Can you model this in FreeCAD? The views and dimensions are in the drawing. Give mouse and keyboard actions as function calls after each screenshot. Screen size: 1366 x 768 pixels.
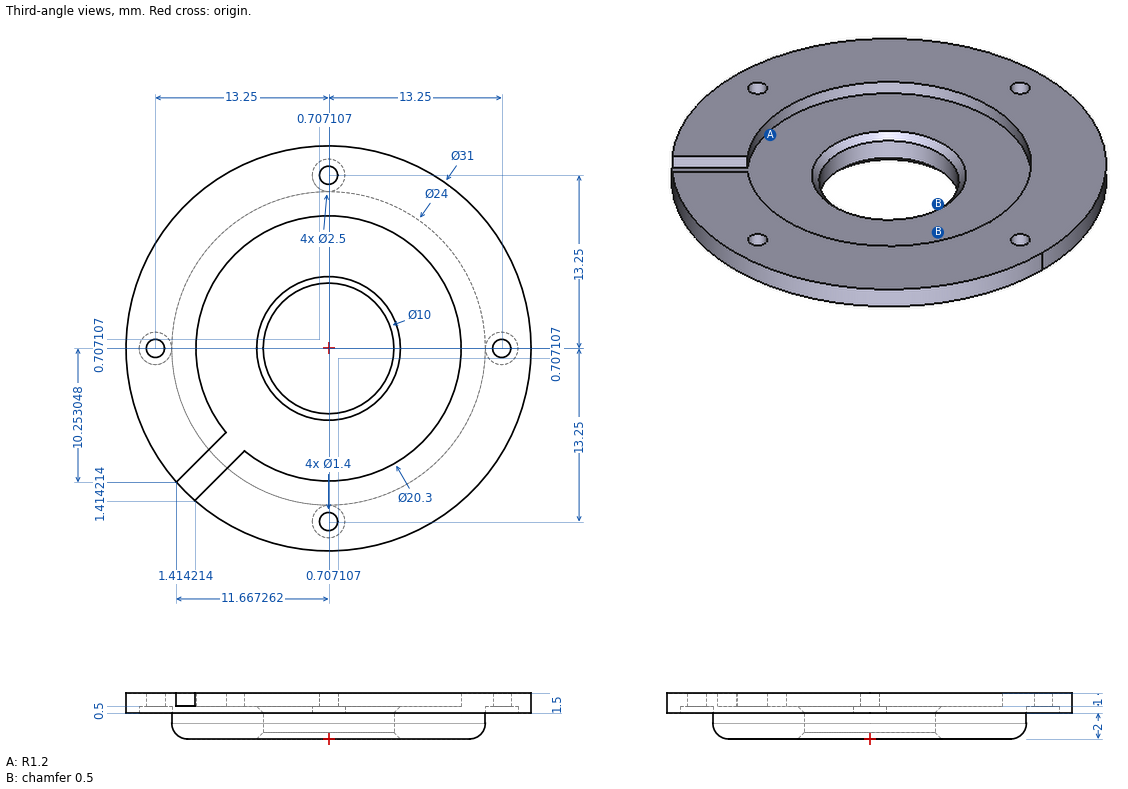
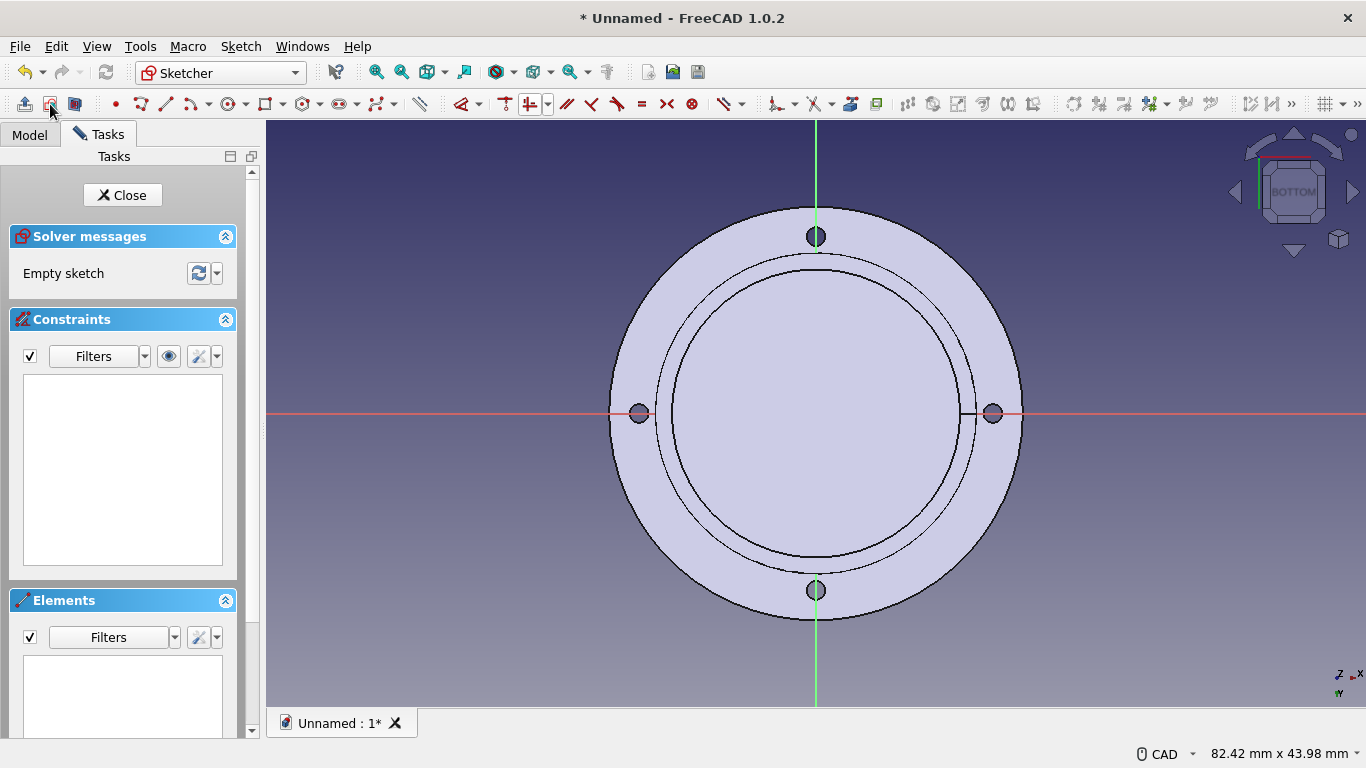
click(228, 104)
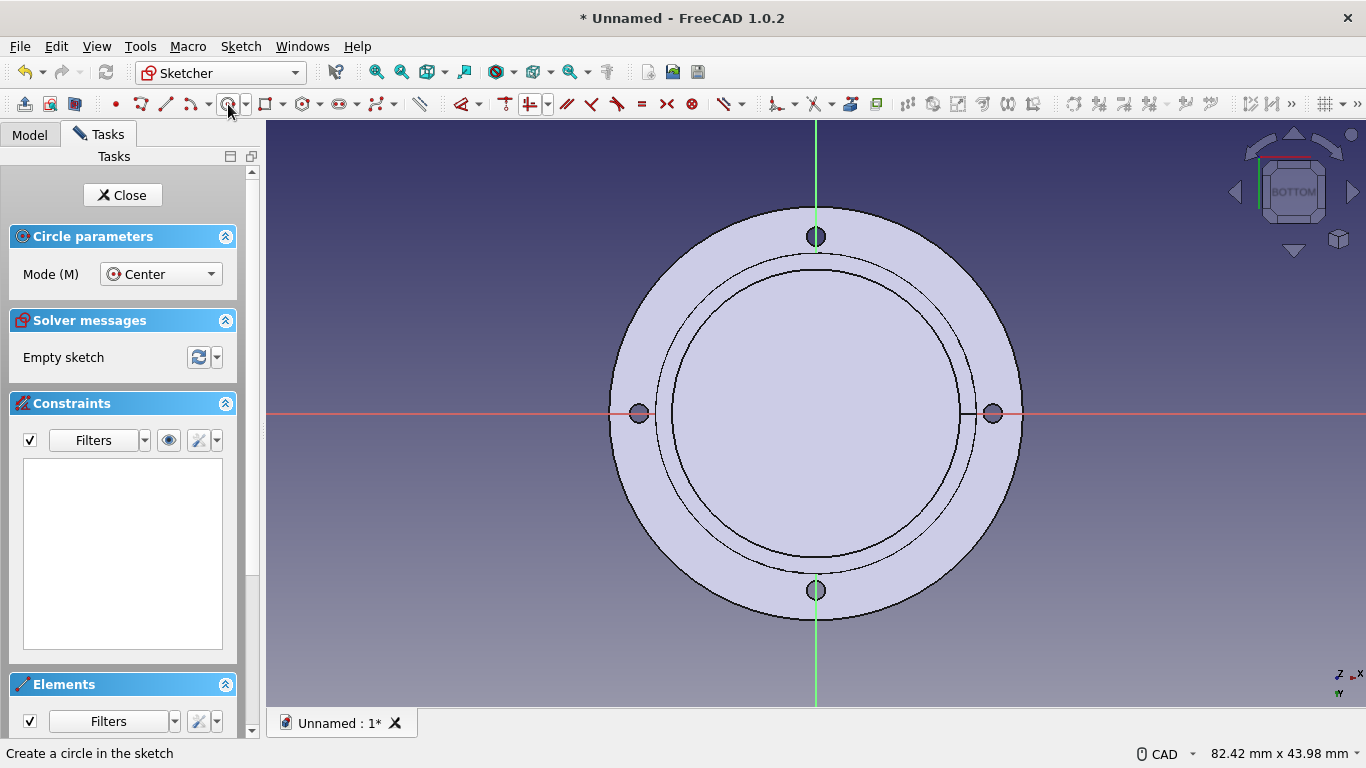
scroll(816, 590, up, 2)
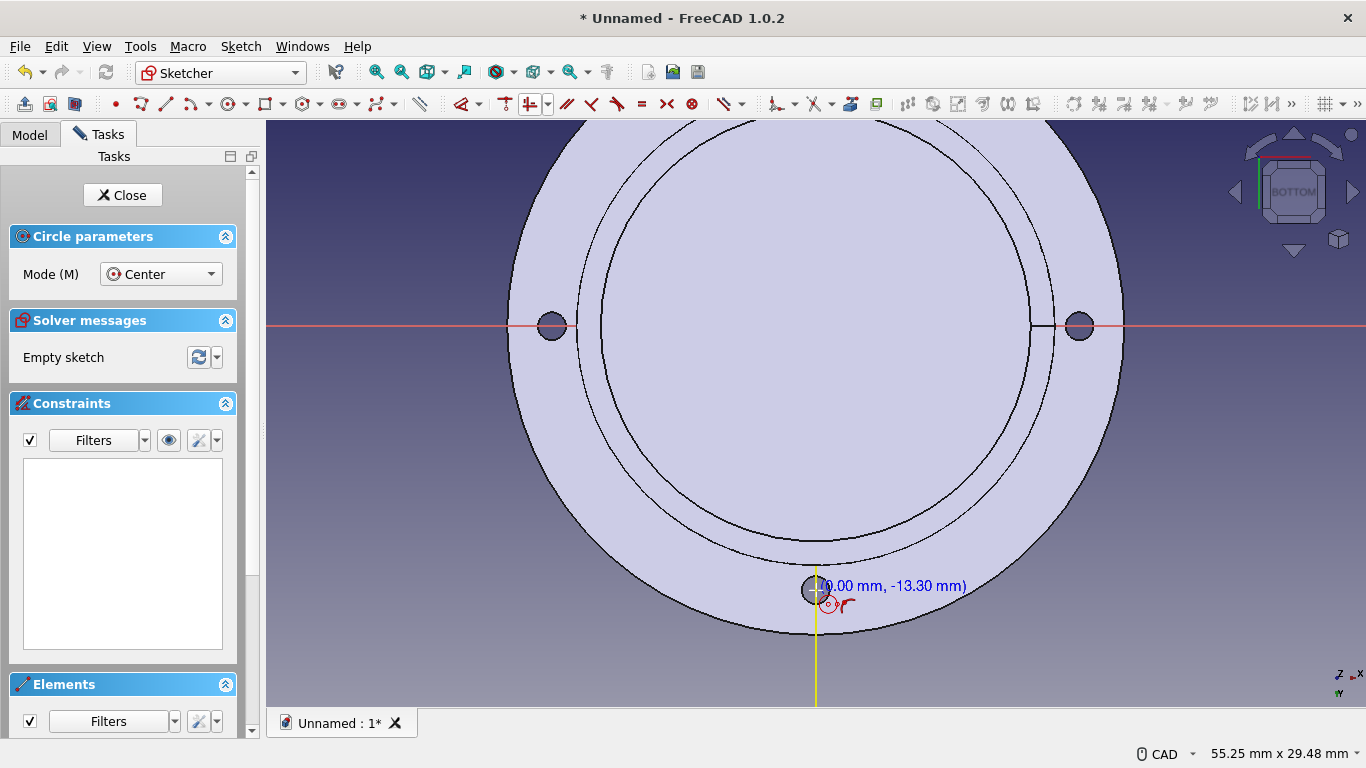
click(816, 590)
move(833, 573)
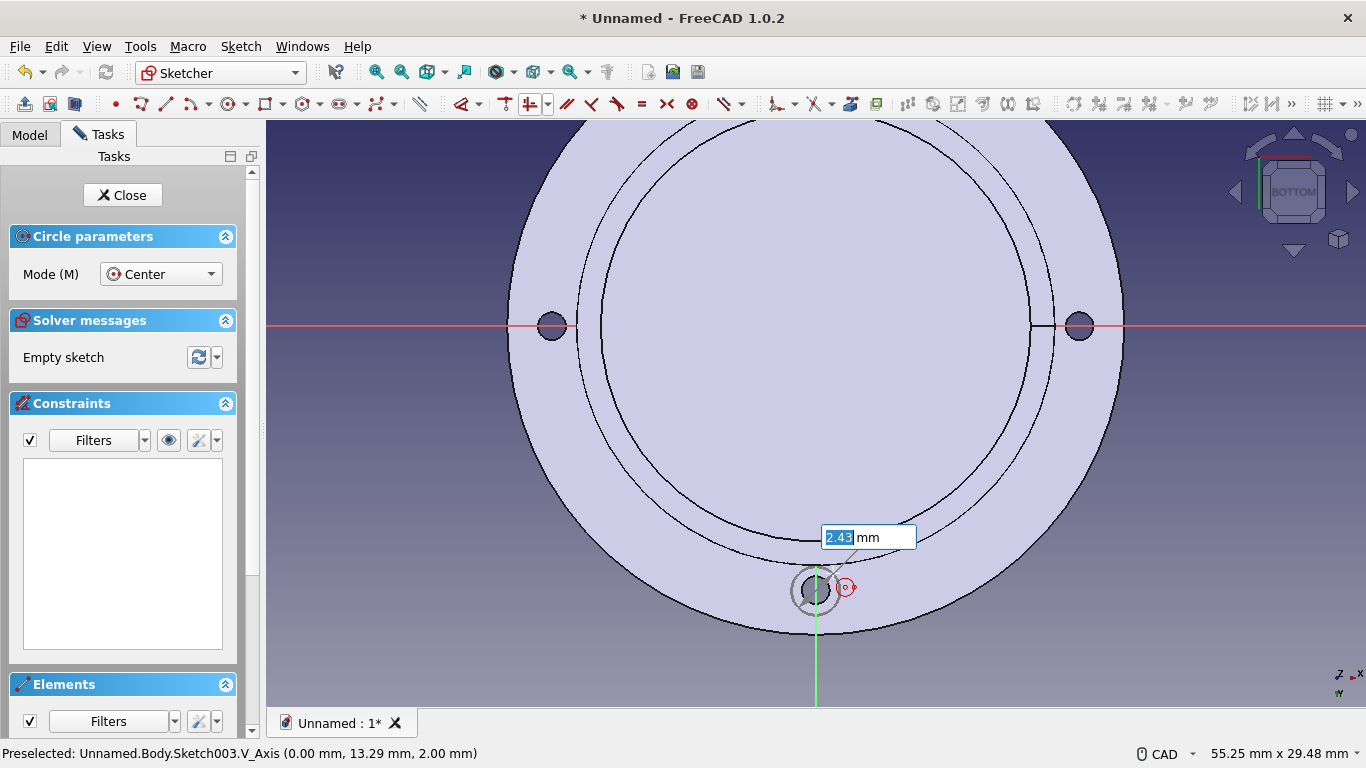
text(2.5)
key(Return)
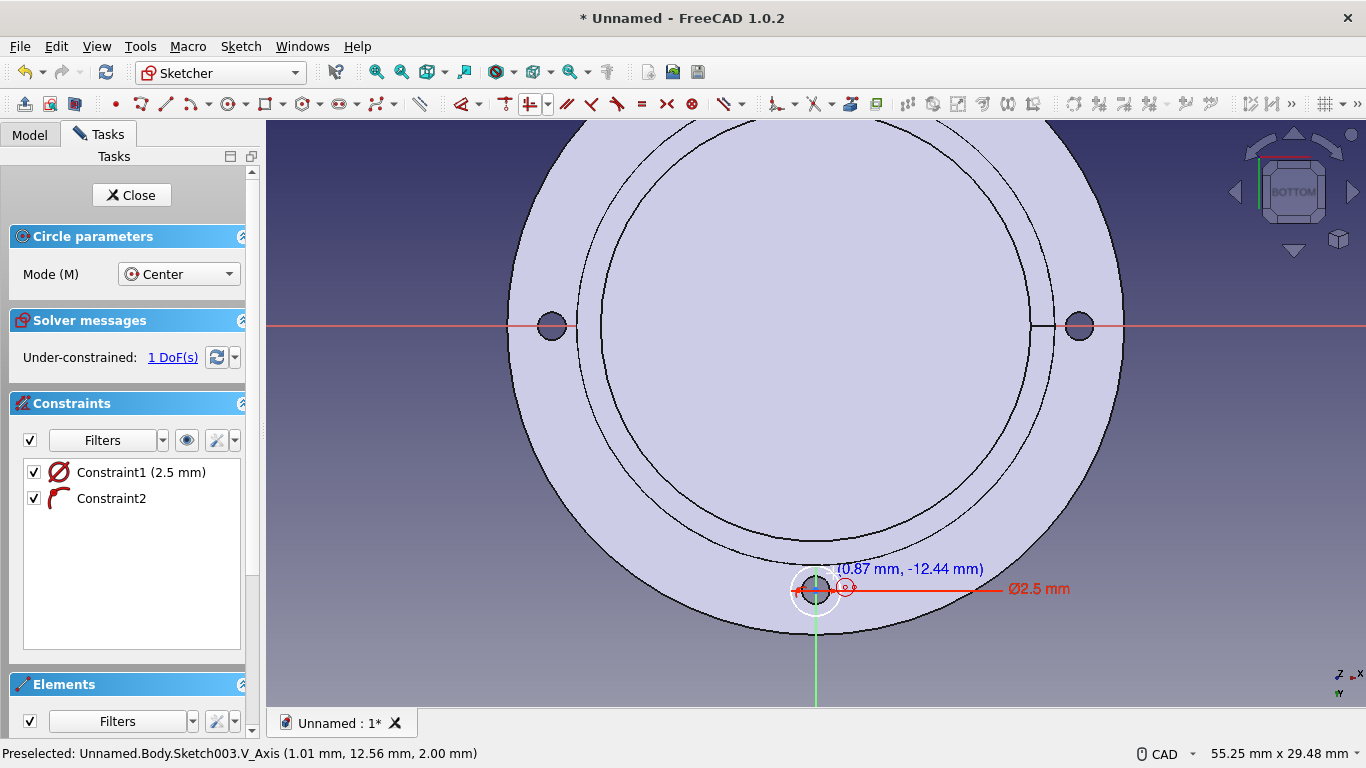
click(552, 326)
move(570, 309)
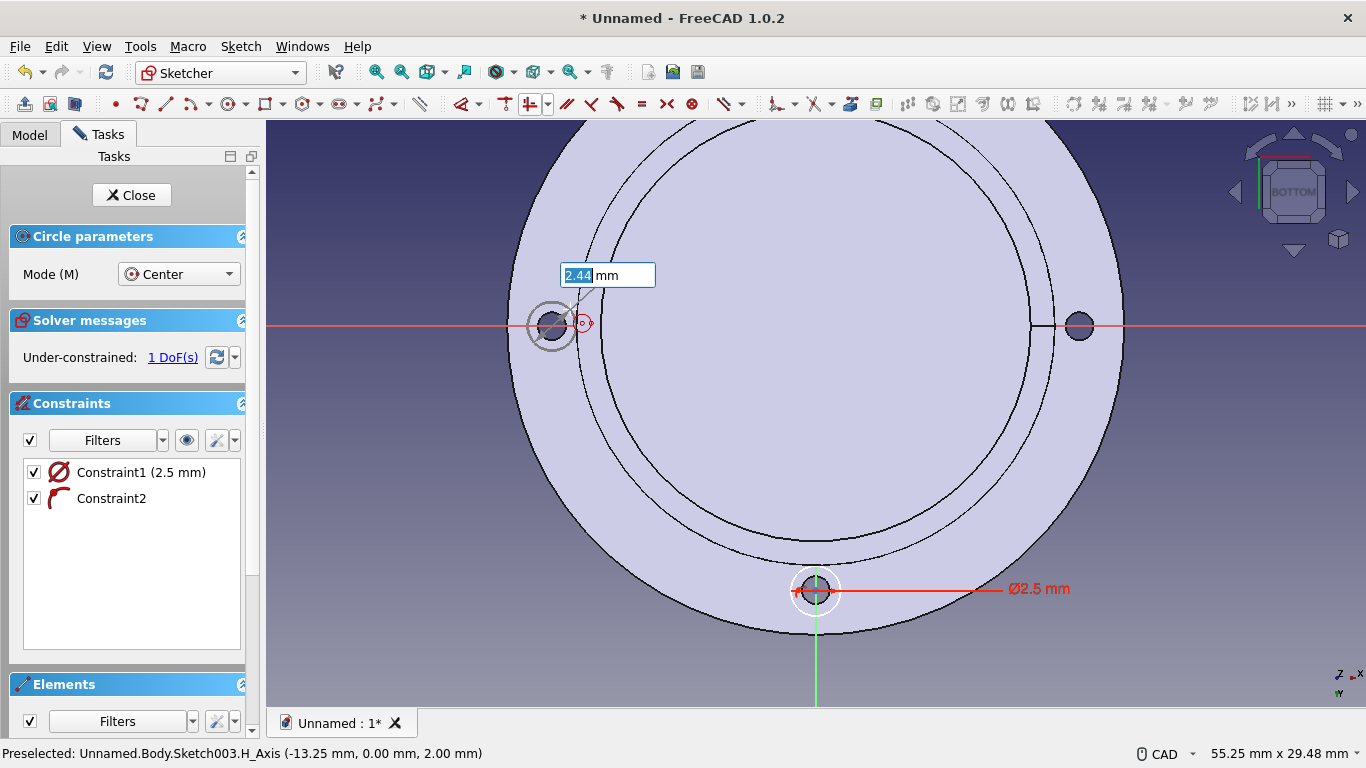
text(2.5)
key(Return)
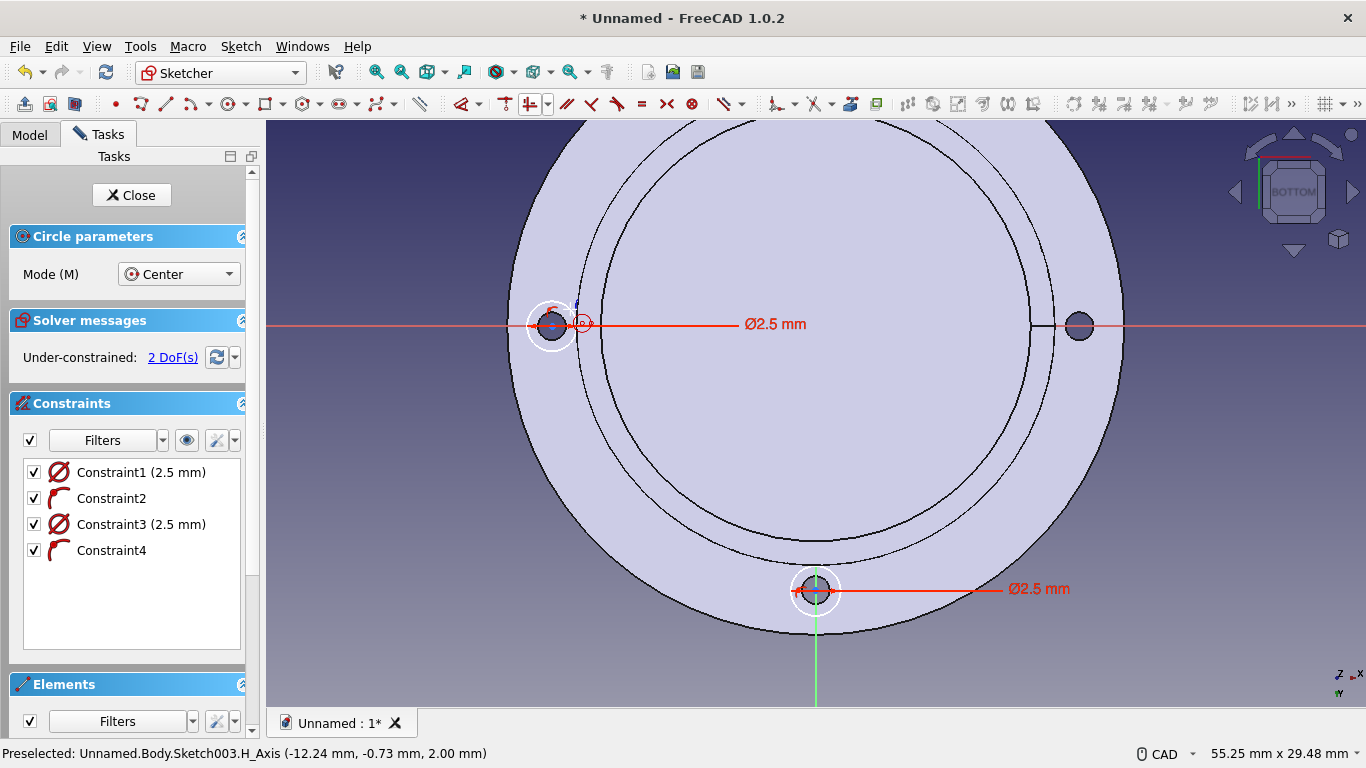
scroll(609, 591, down, 2)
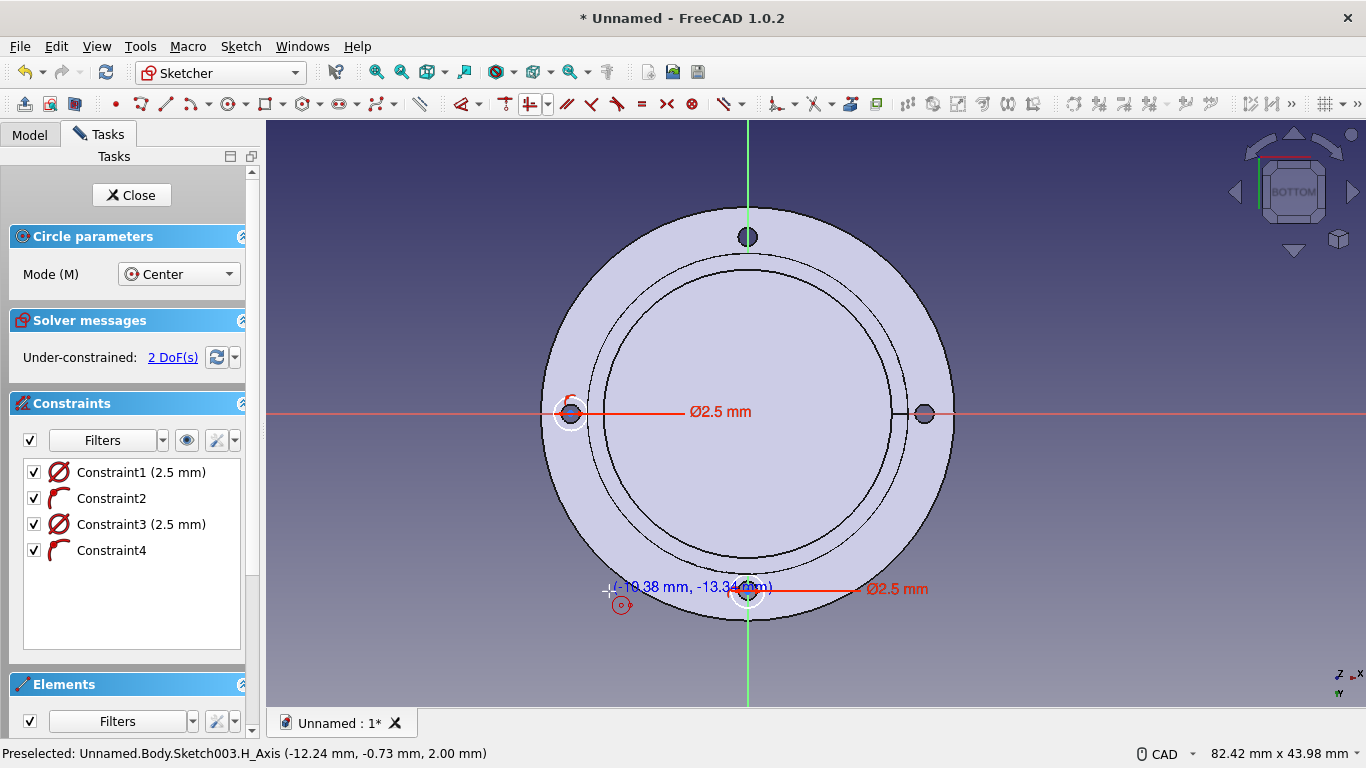
scroll(748, 237, up, 2)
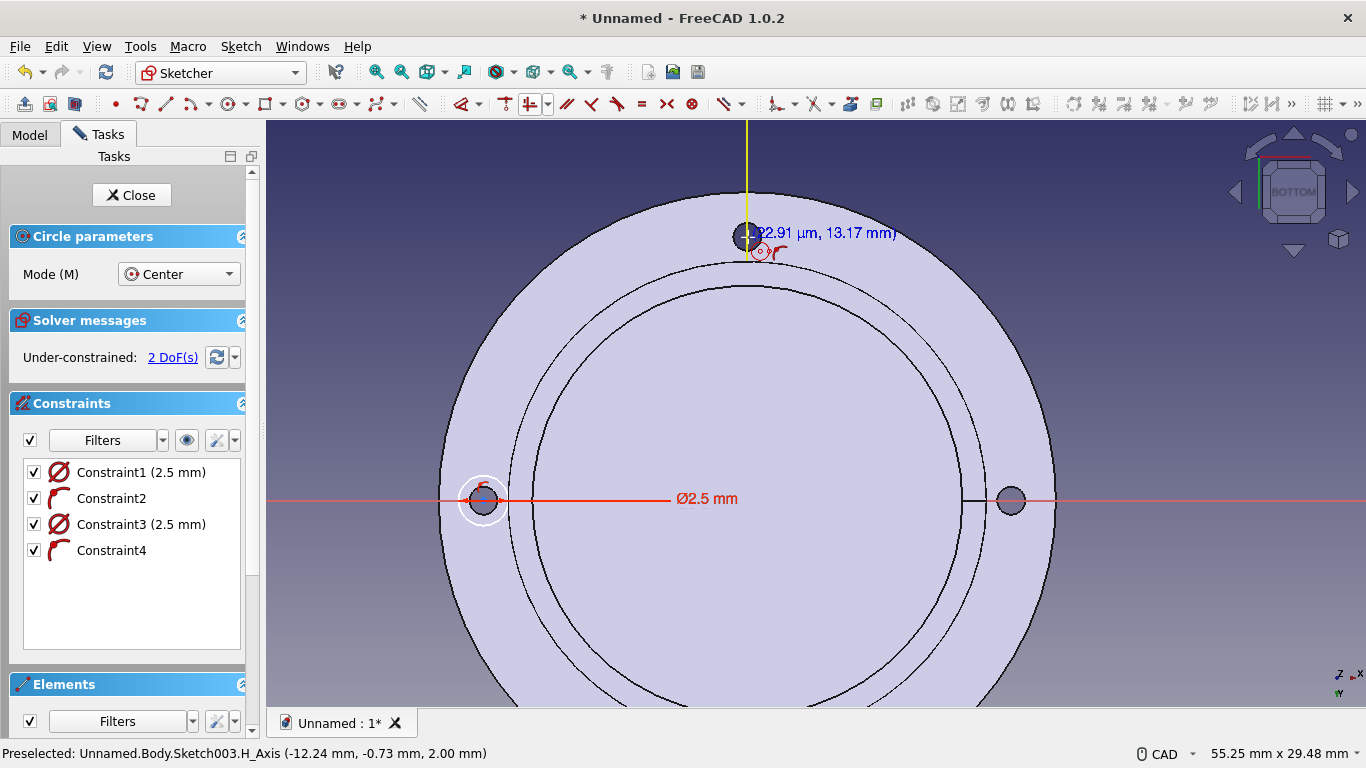
click(747, 237)
move(765, 219)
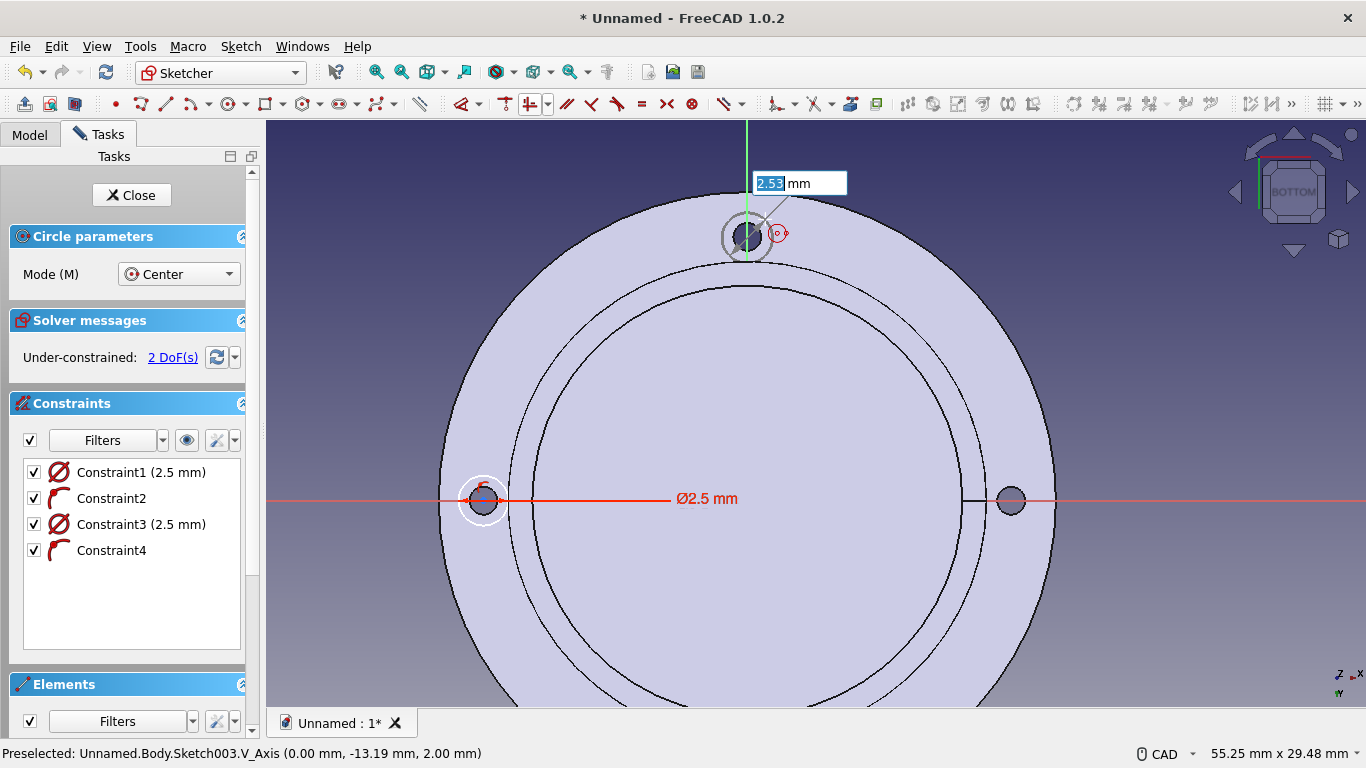
text(2.5)
key(Return)